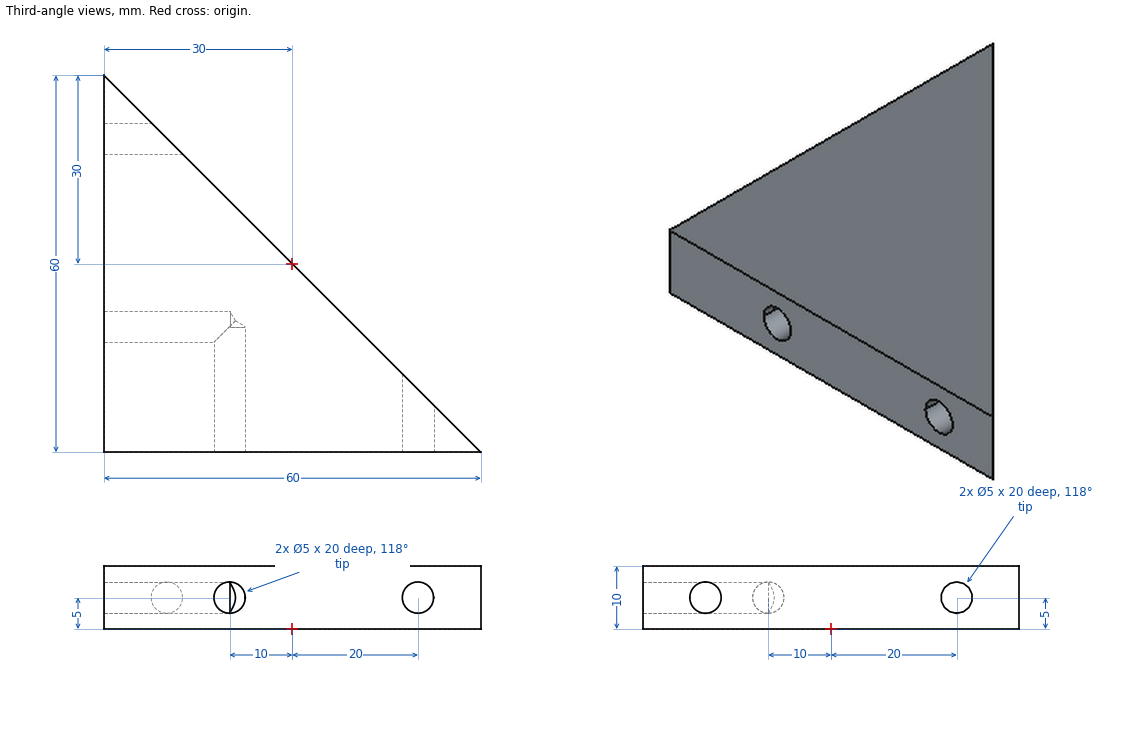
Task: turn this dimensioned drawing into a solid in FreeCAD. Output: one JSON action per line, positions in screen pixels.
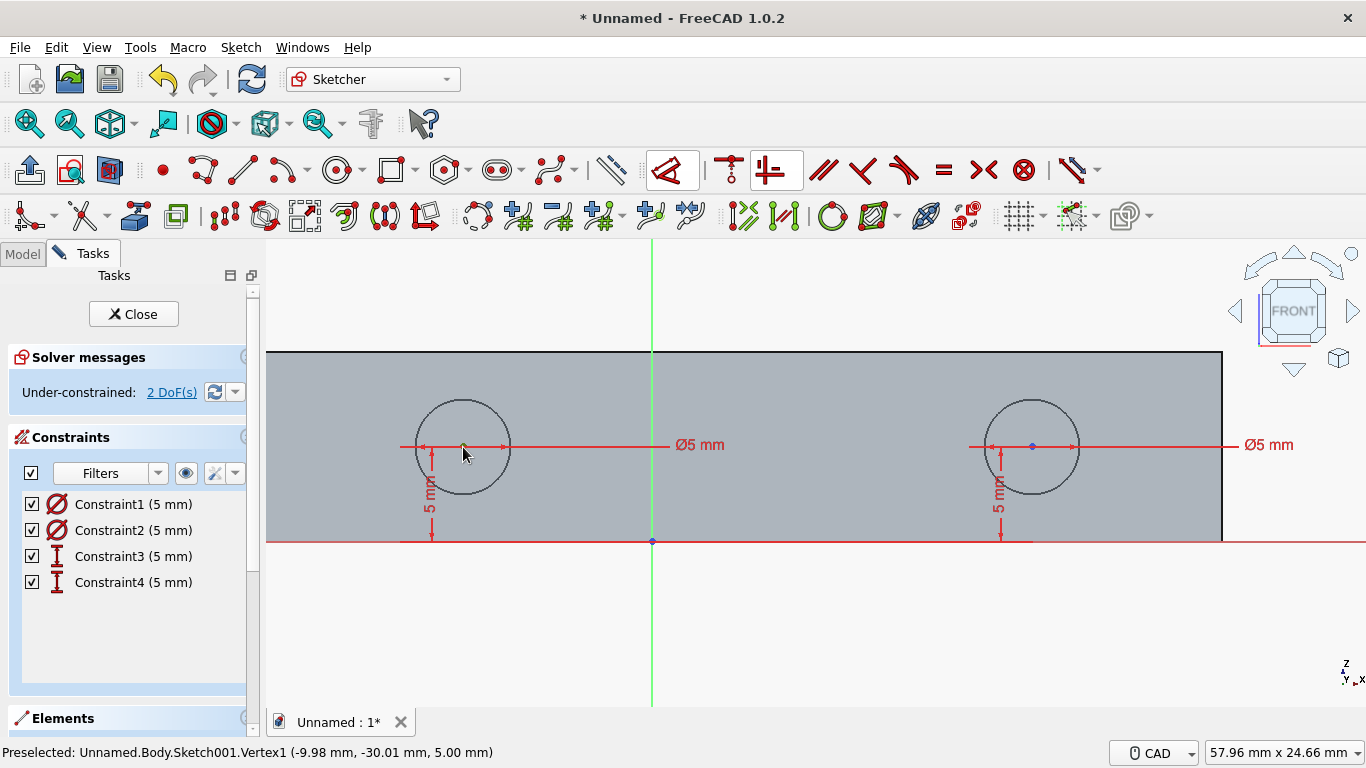
{"action": "key", "text": "l"}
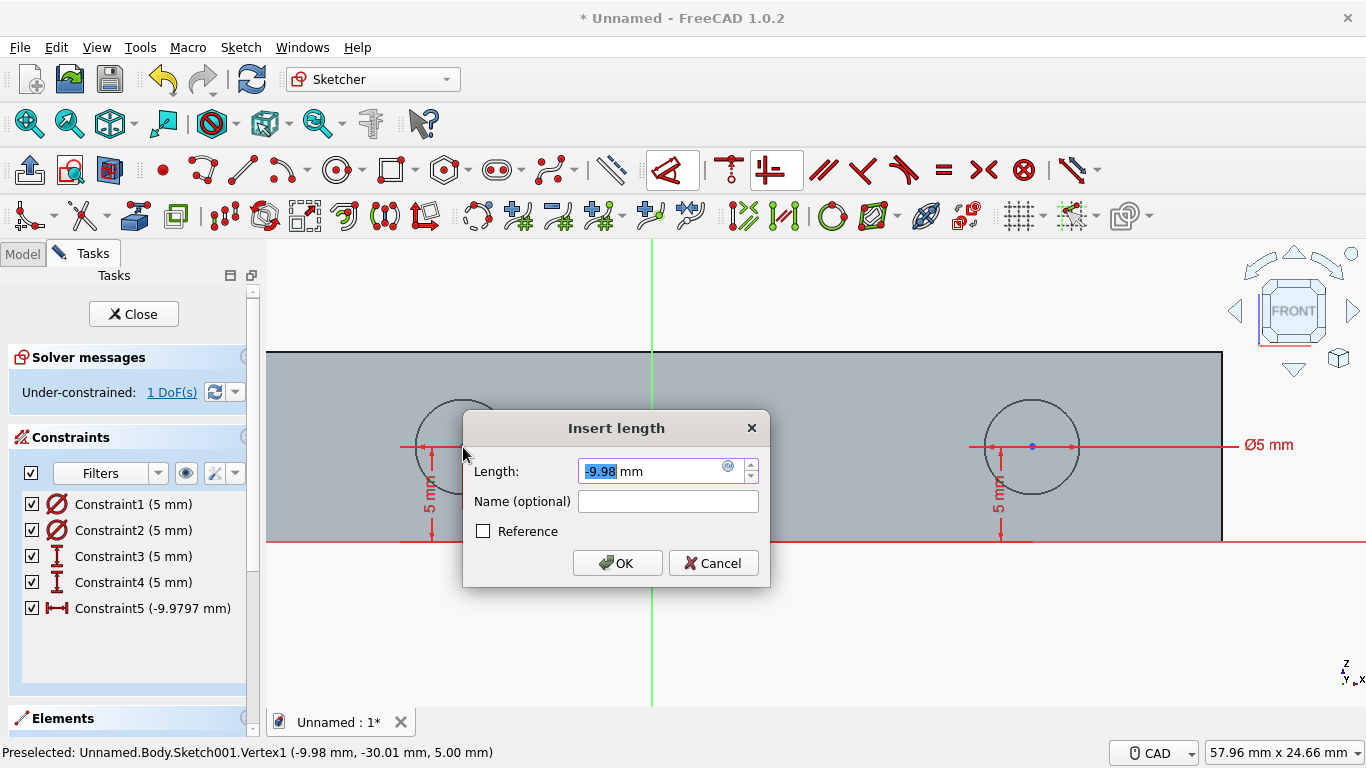
{"action": "type", "text": "-10"}
{"action": "key", "text": "Return"}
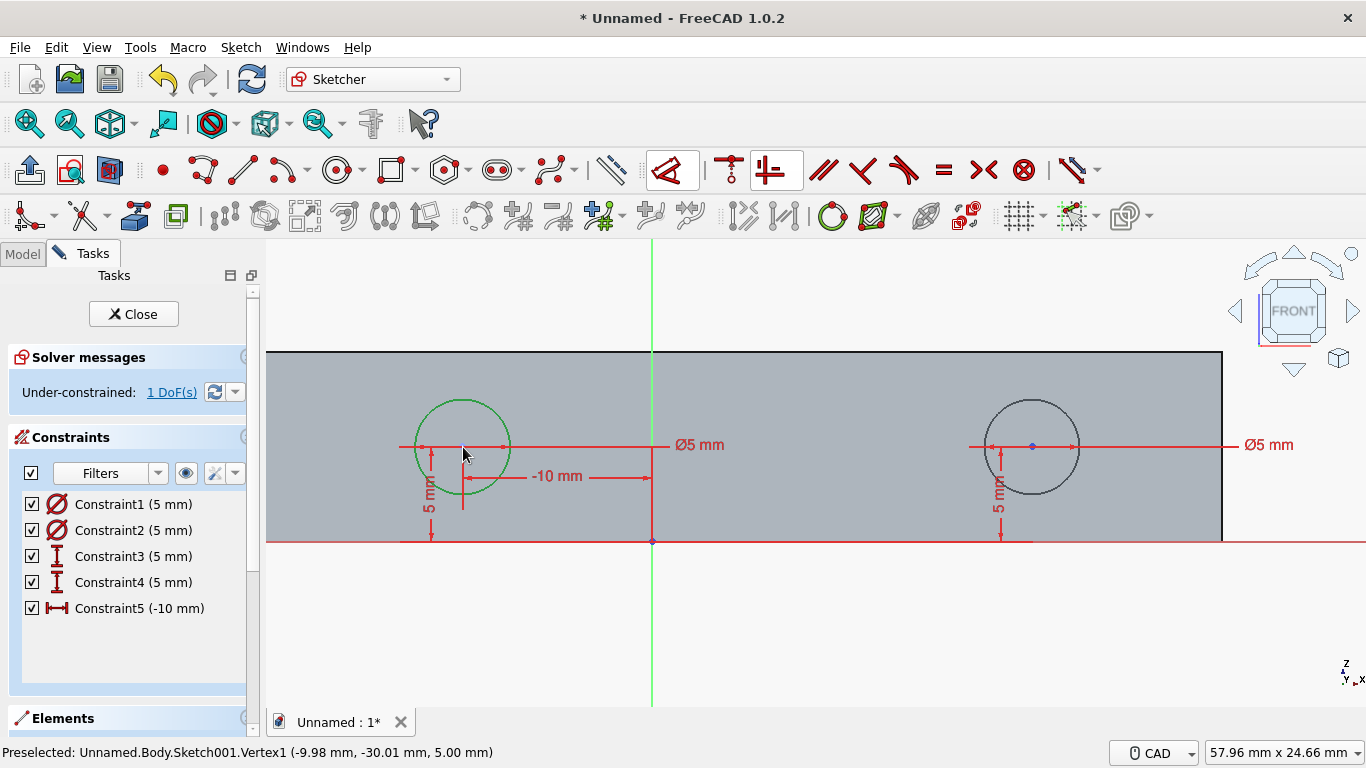
{"action": "left_click", "coordinate": [1032, 447]}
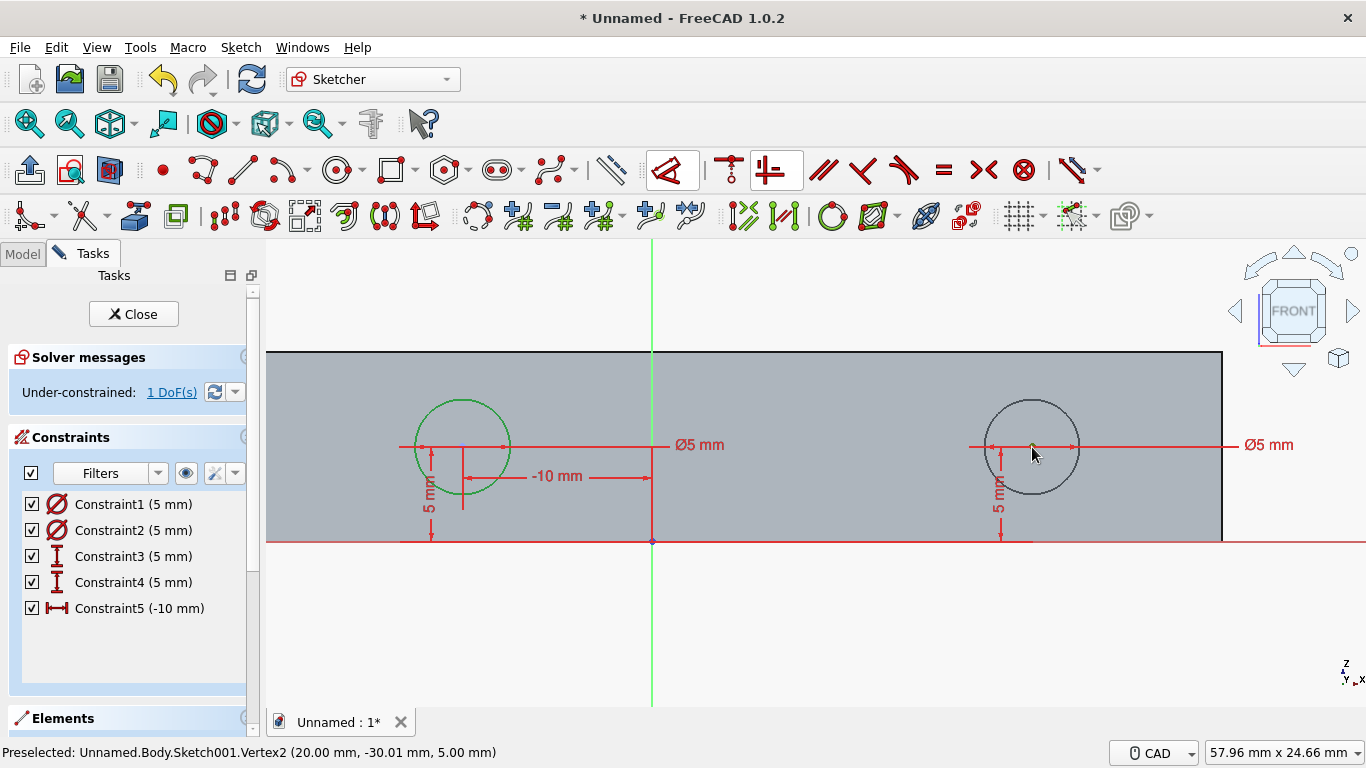
{"action": "key", "text": "l"}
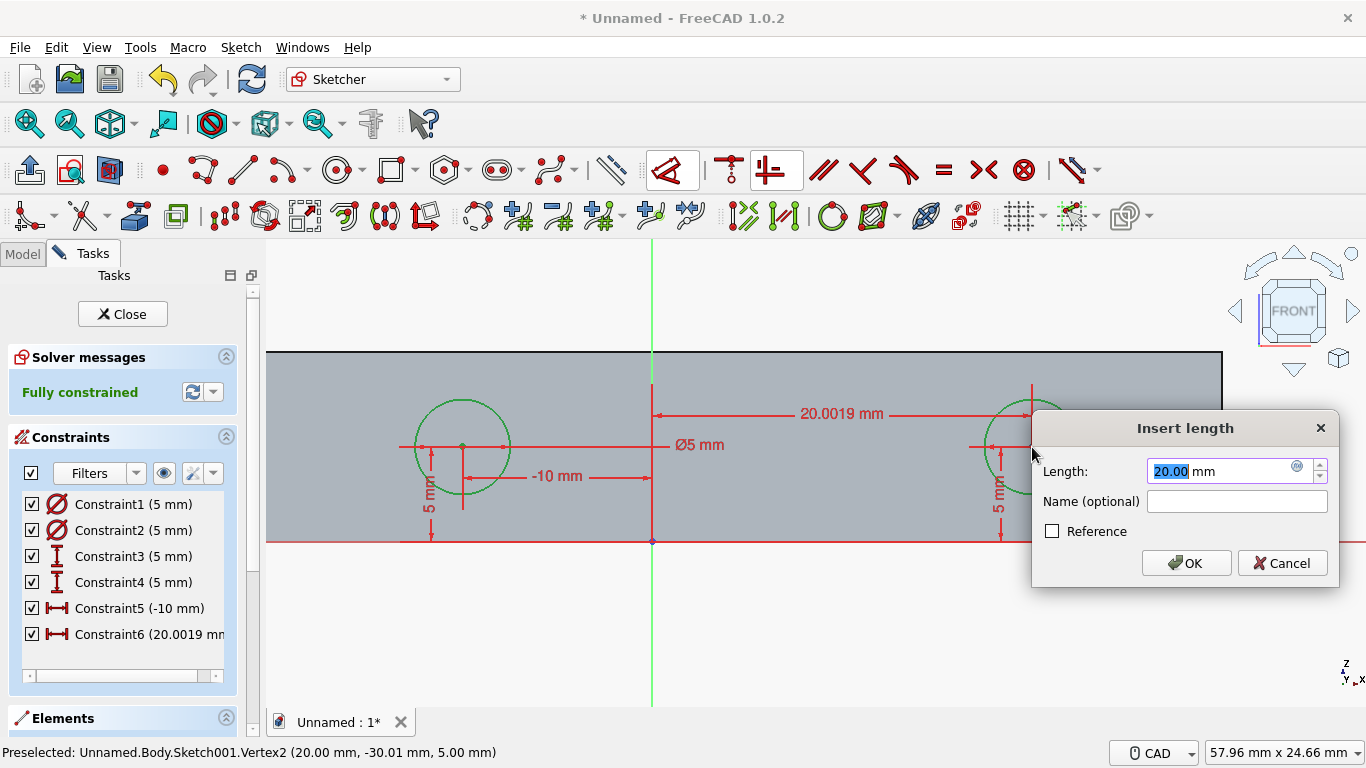
{"action": "type", "text": "20"}
{"action": "key", "text": "Return"}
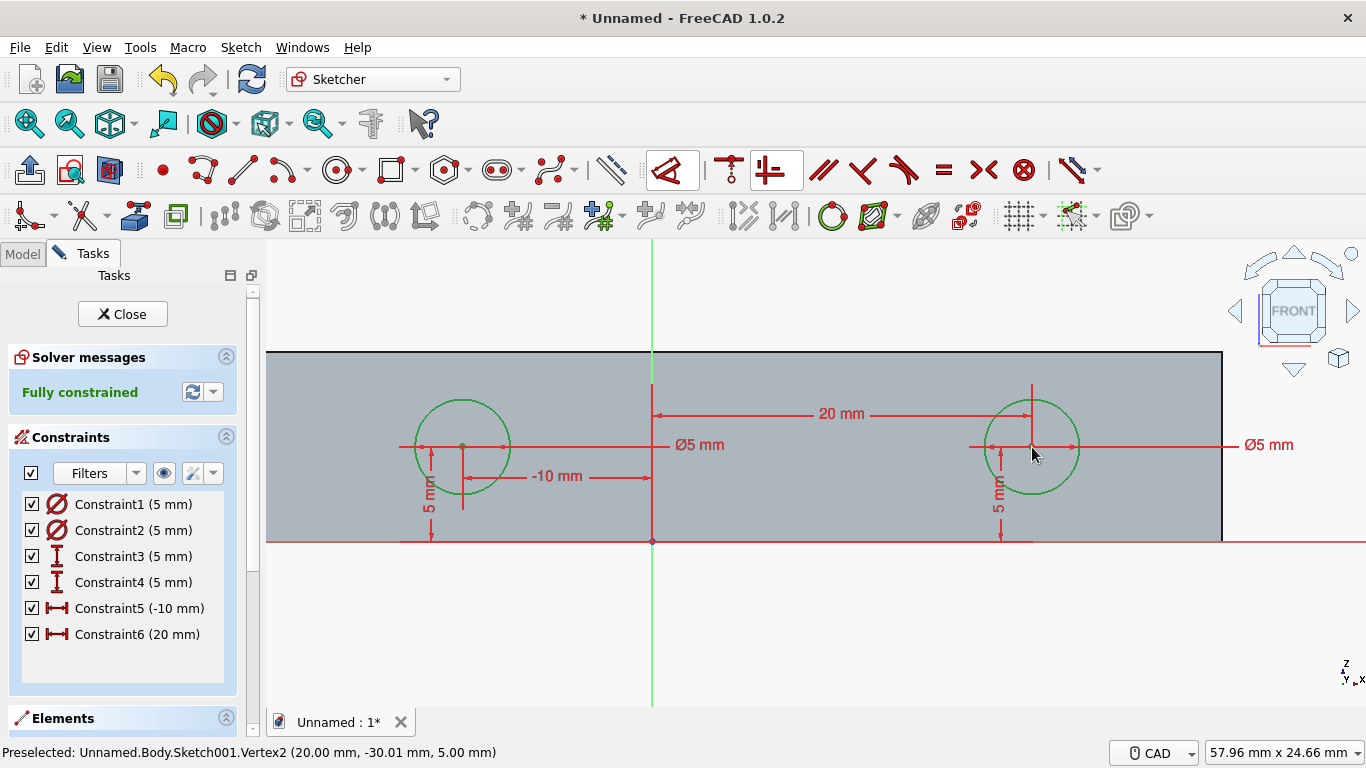
{"action": "left_click", "coordinate": [123, 314]}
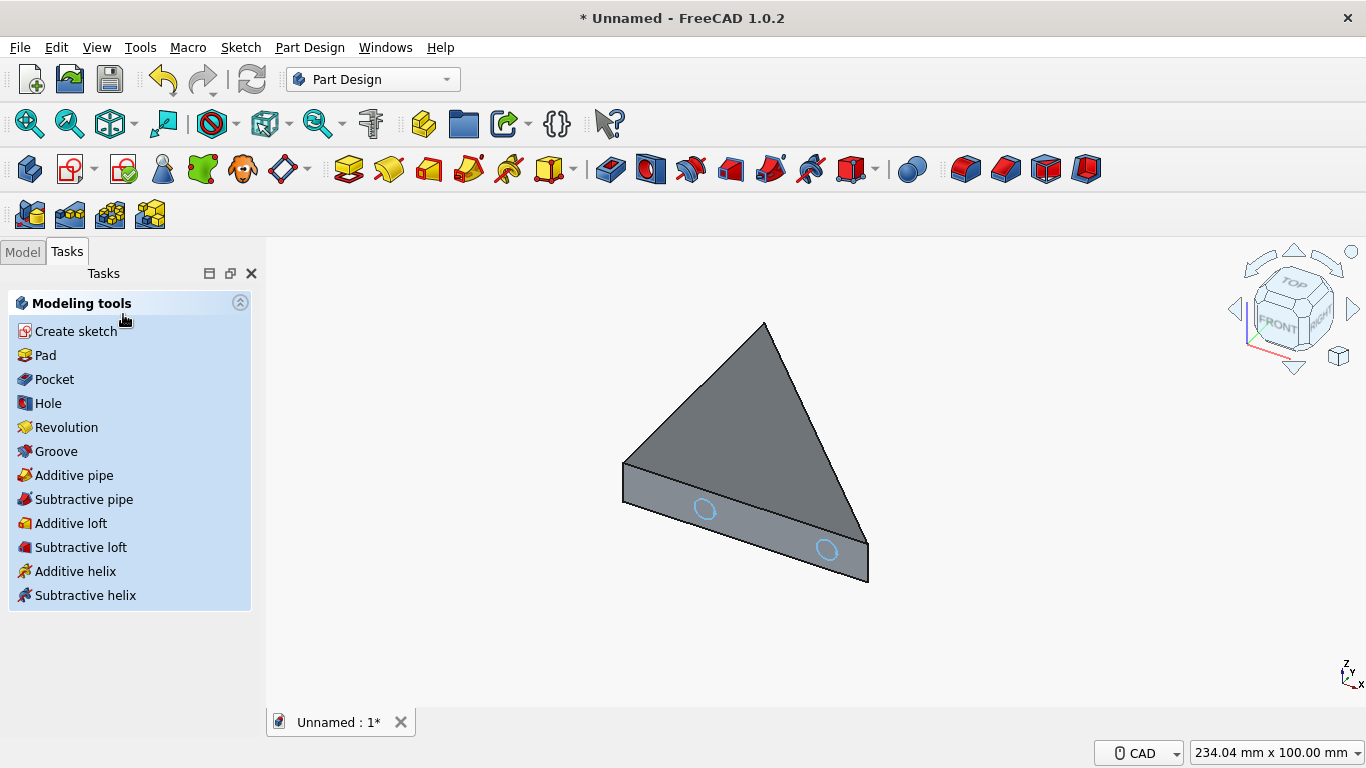
{"action": "left_click", "coordinate": [652, 170]}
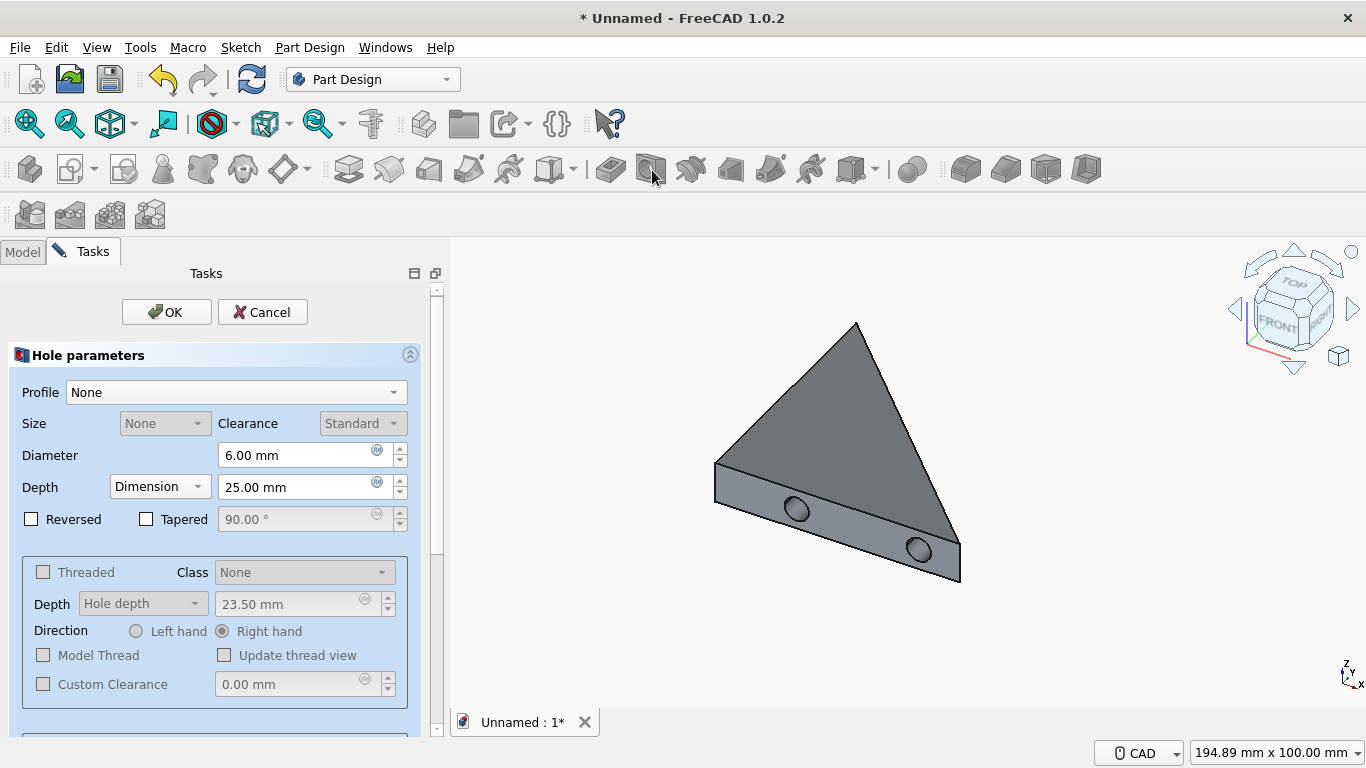
{"action": "triple_click", "coordinate": [305, 455]}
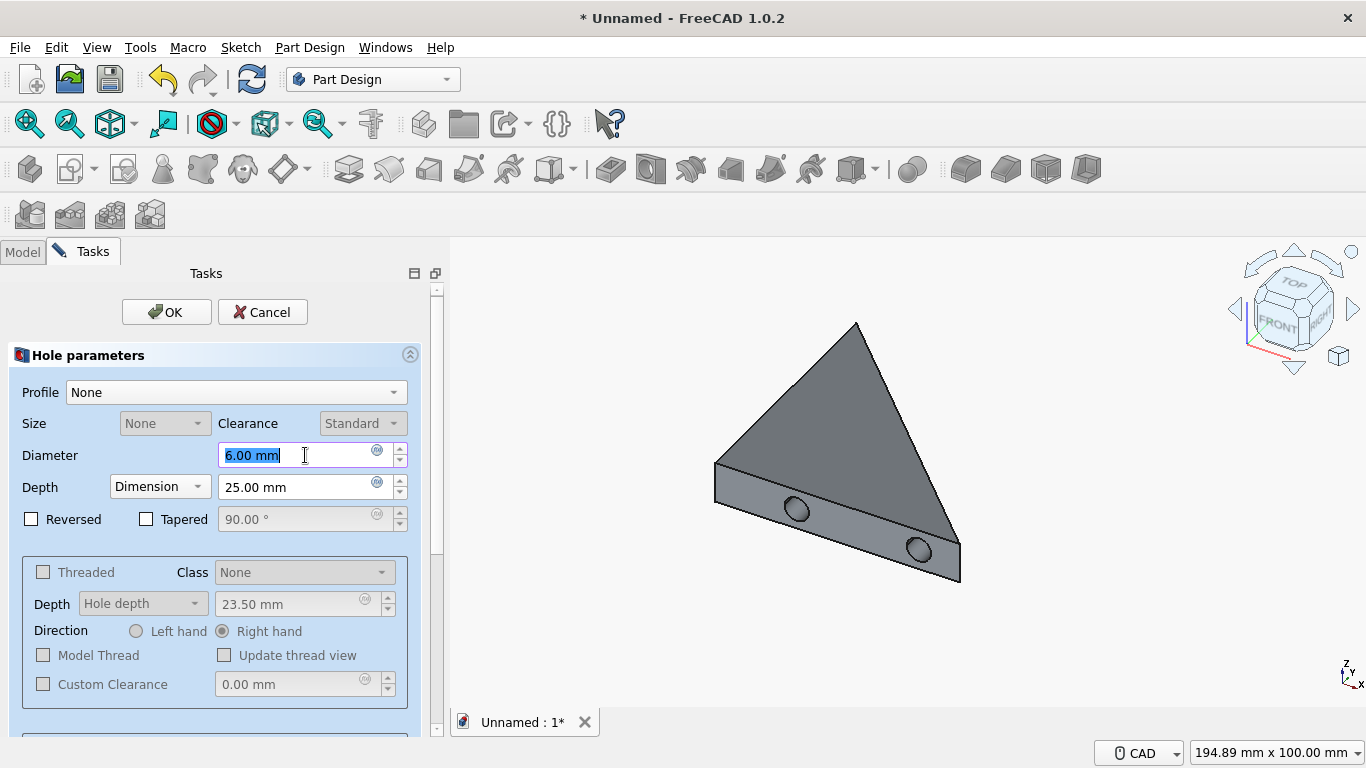
{"action": "type", "text": "5"}
{"action": "key", "text": "Tab"}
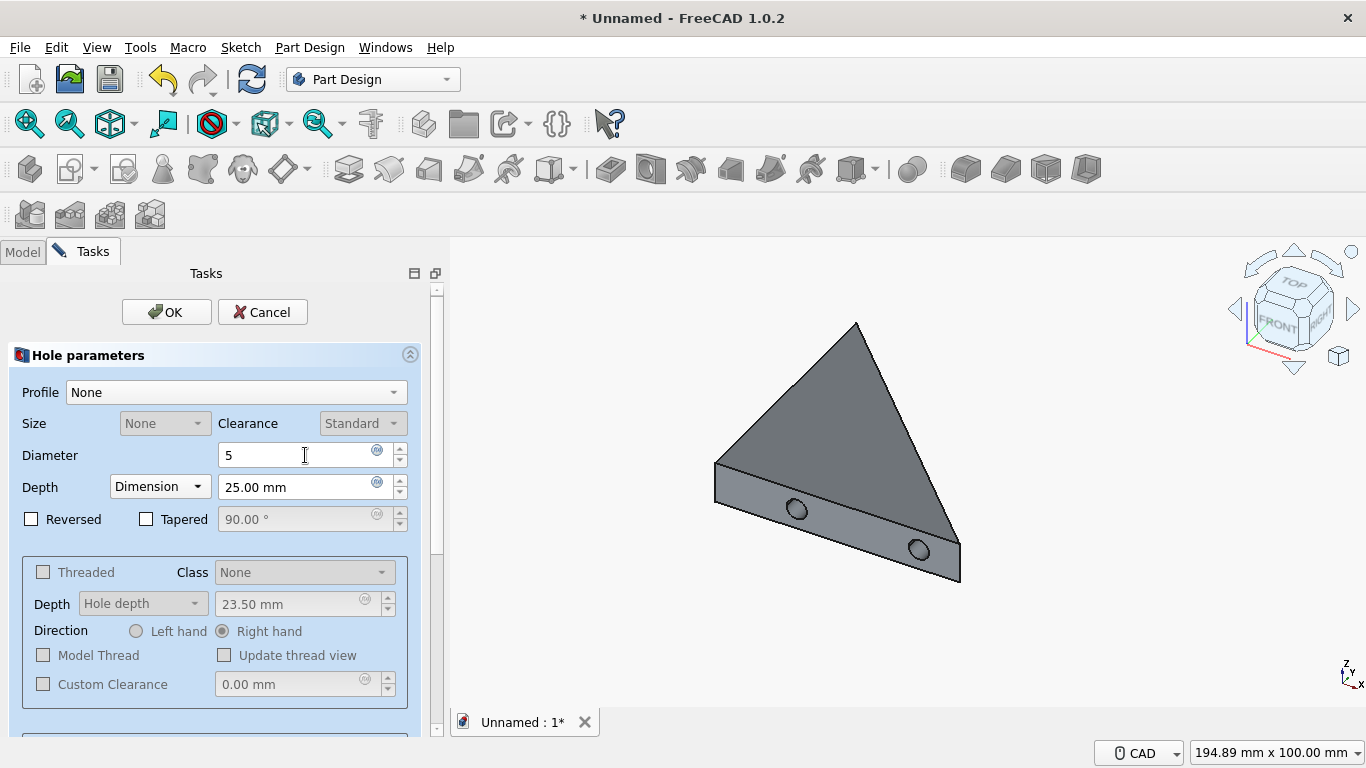
{"action": "triple_click", "coordinate": [305, 487]}